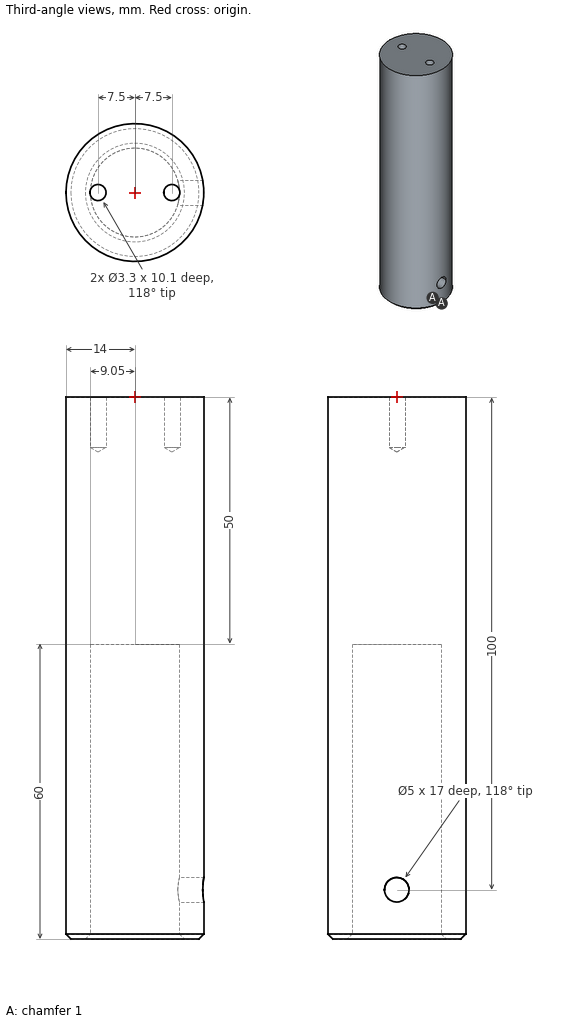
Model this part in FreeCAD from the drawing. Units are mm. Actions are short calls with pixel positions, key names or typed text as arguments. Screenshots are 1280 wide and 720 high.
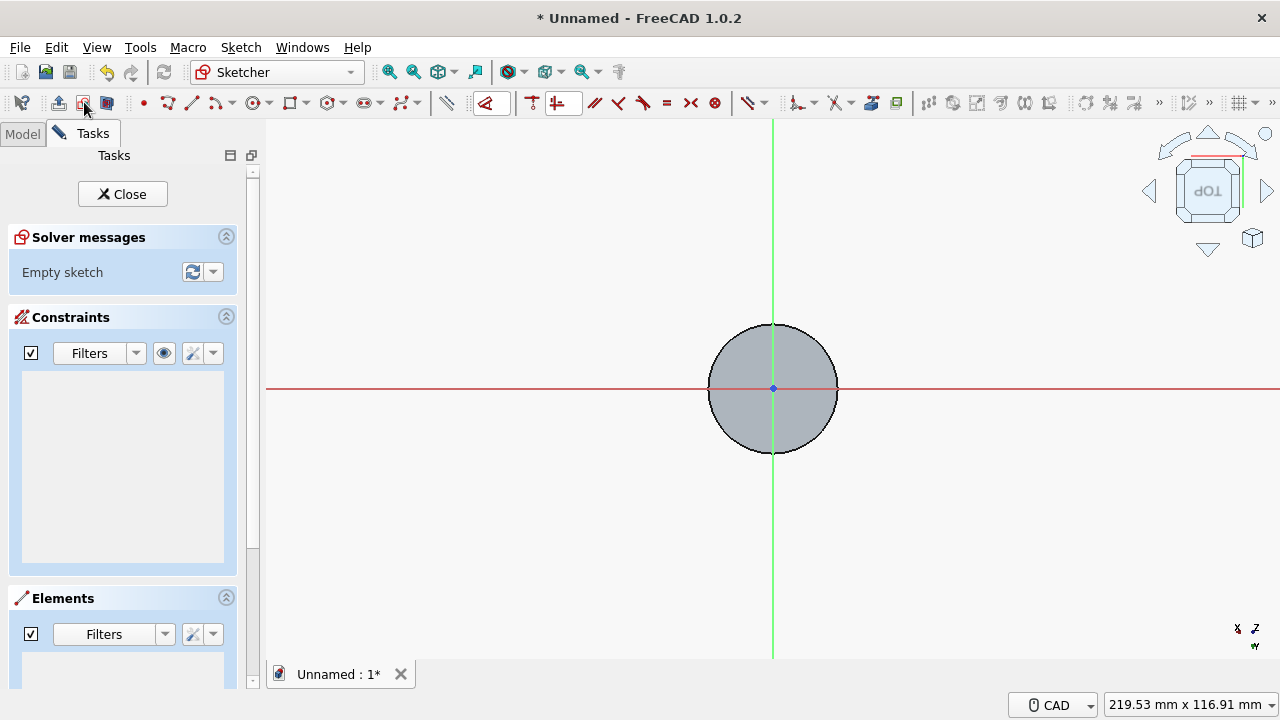
scroll(784, 389, up, 10)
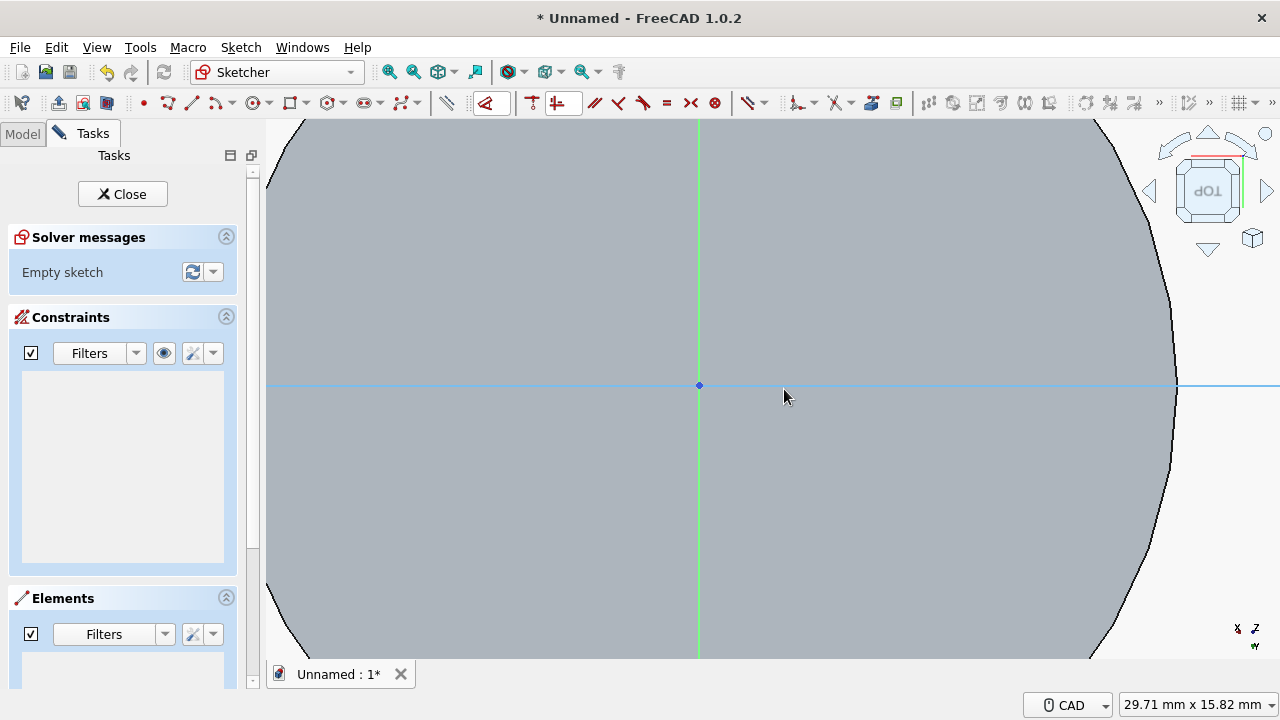
click(254, 104)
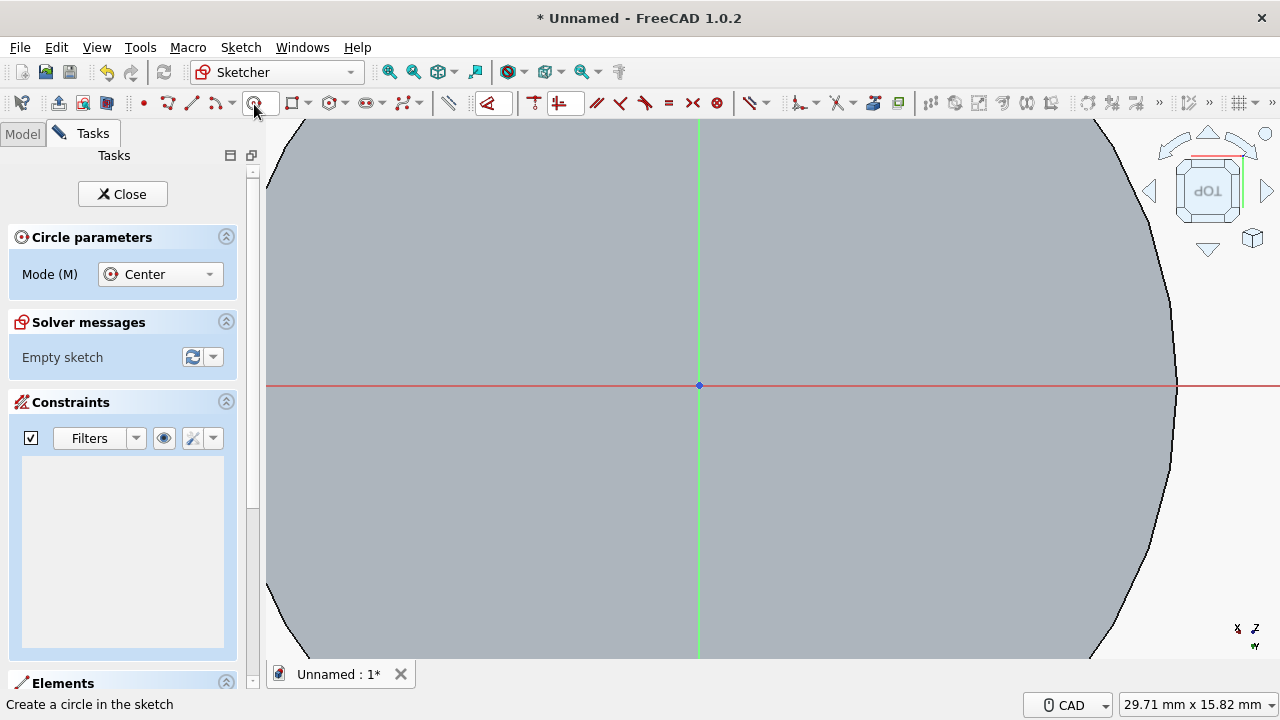
click(955, 386)
click(995, 346)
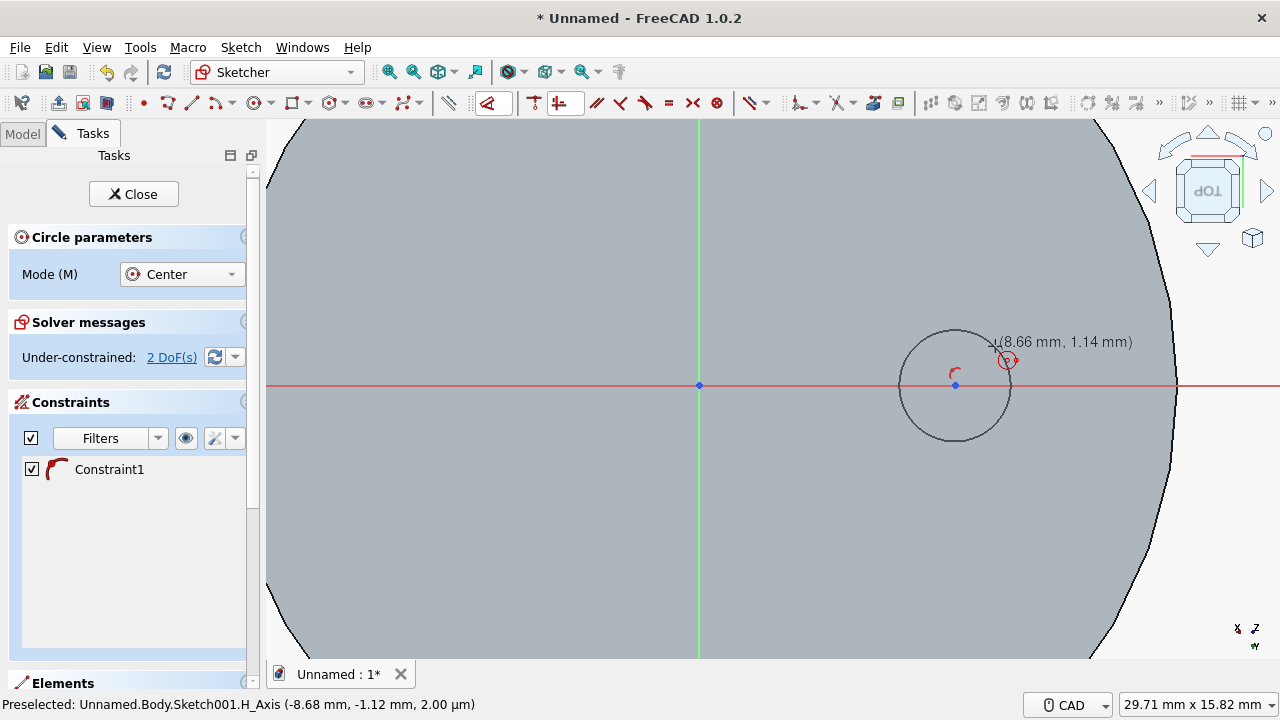
click(443, 386)
click(483, 346)
key(Escape)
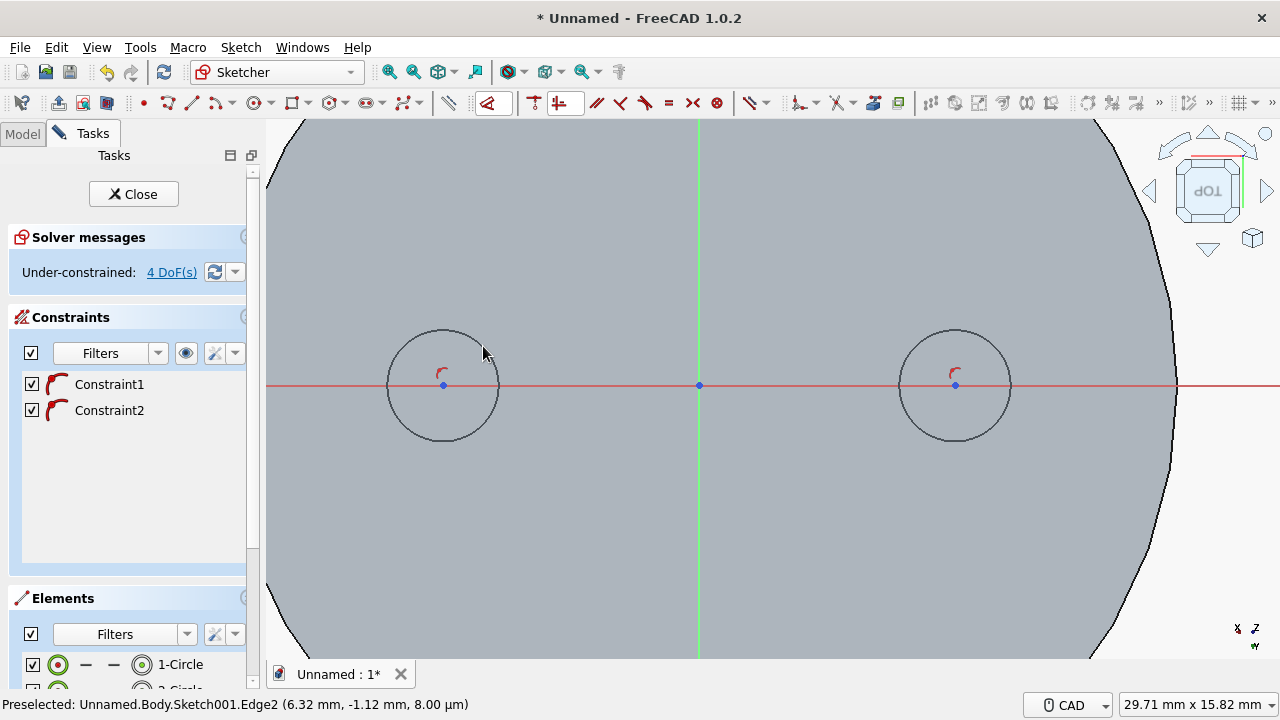
click(994, 346)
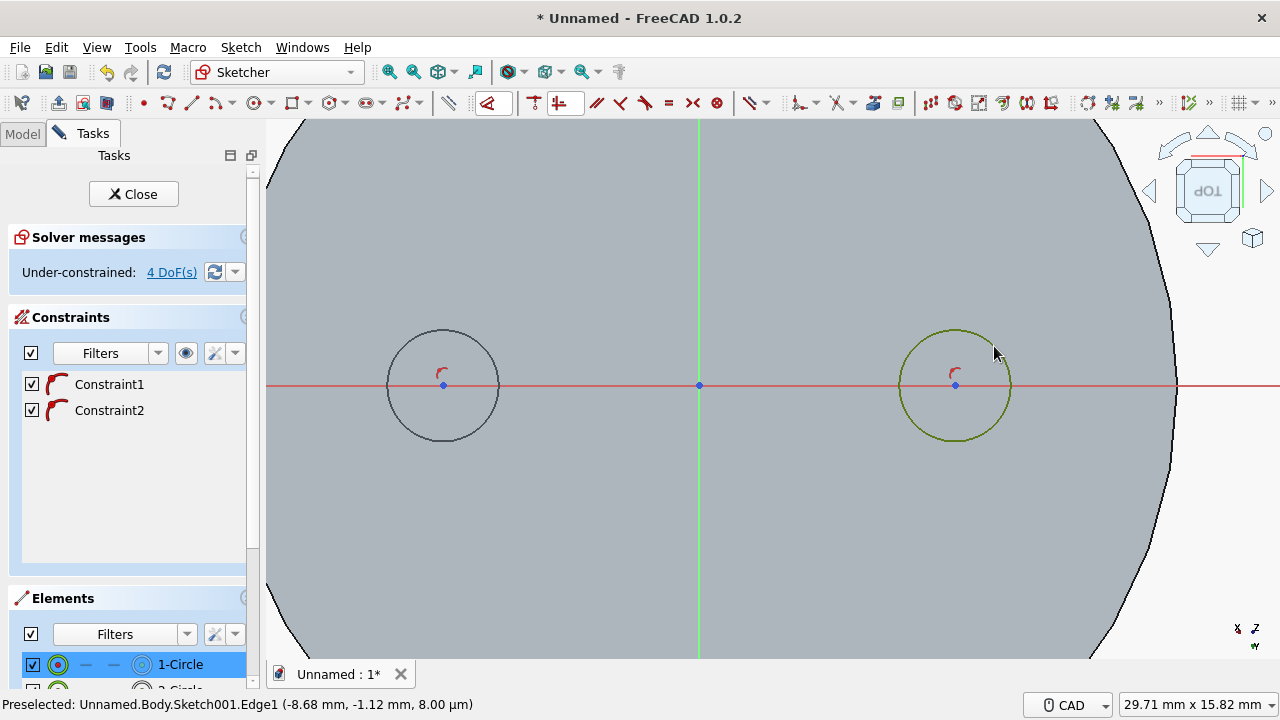
click(482, 346)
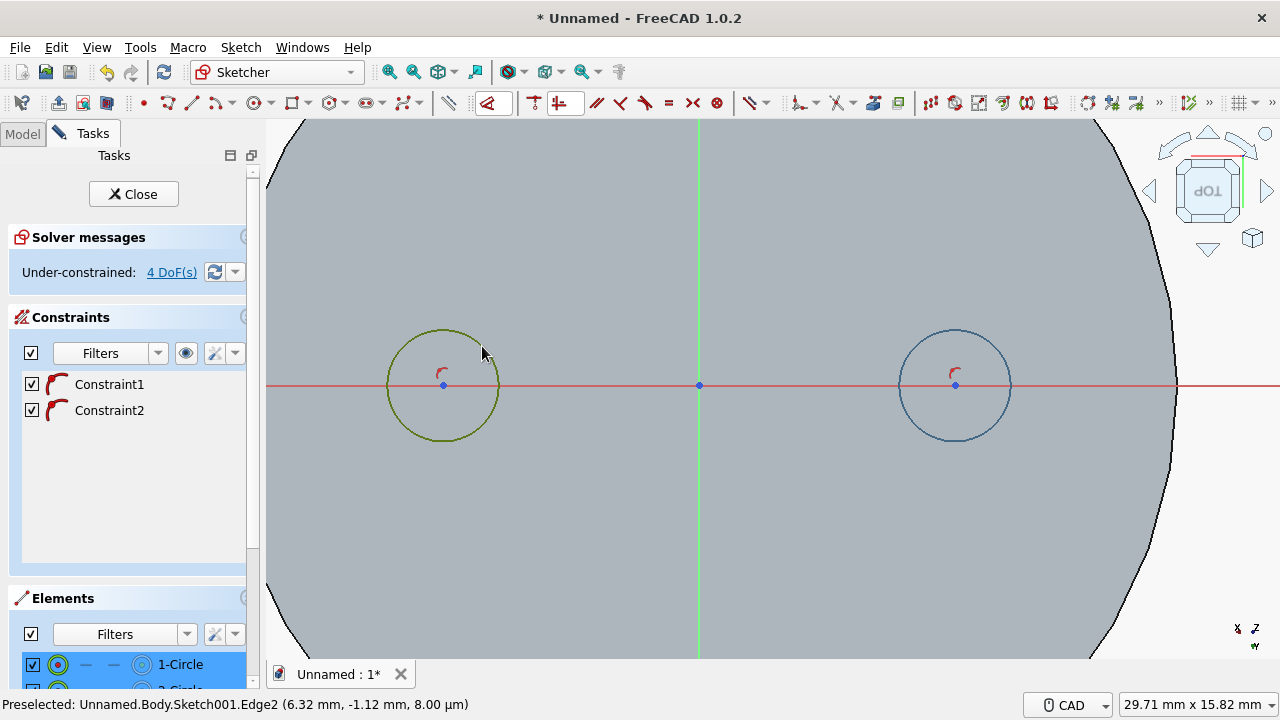
click(670, 104)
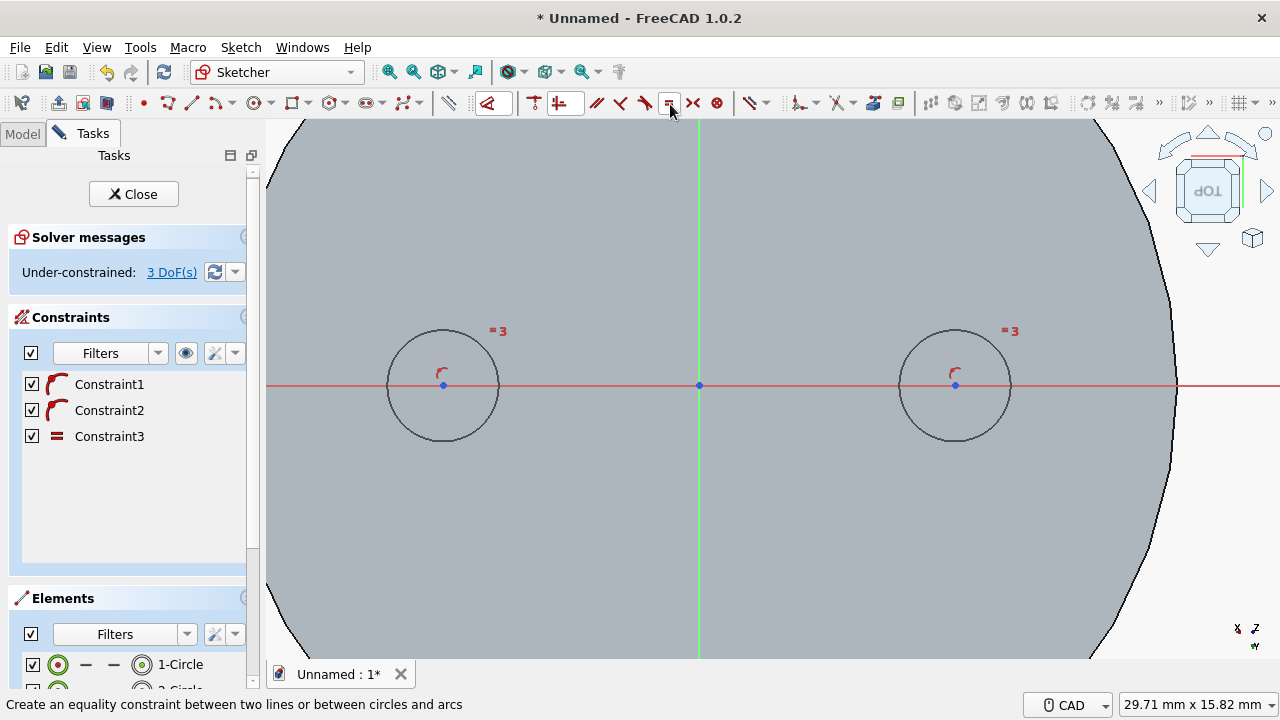
click(994, 346)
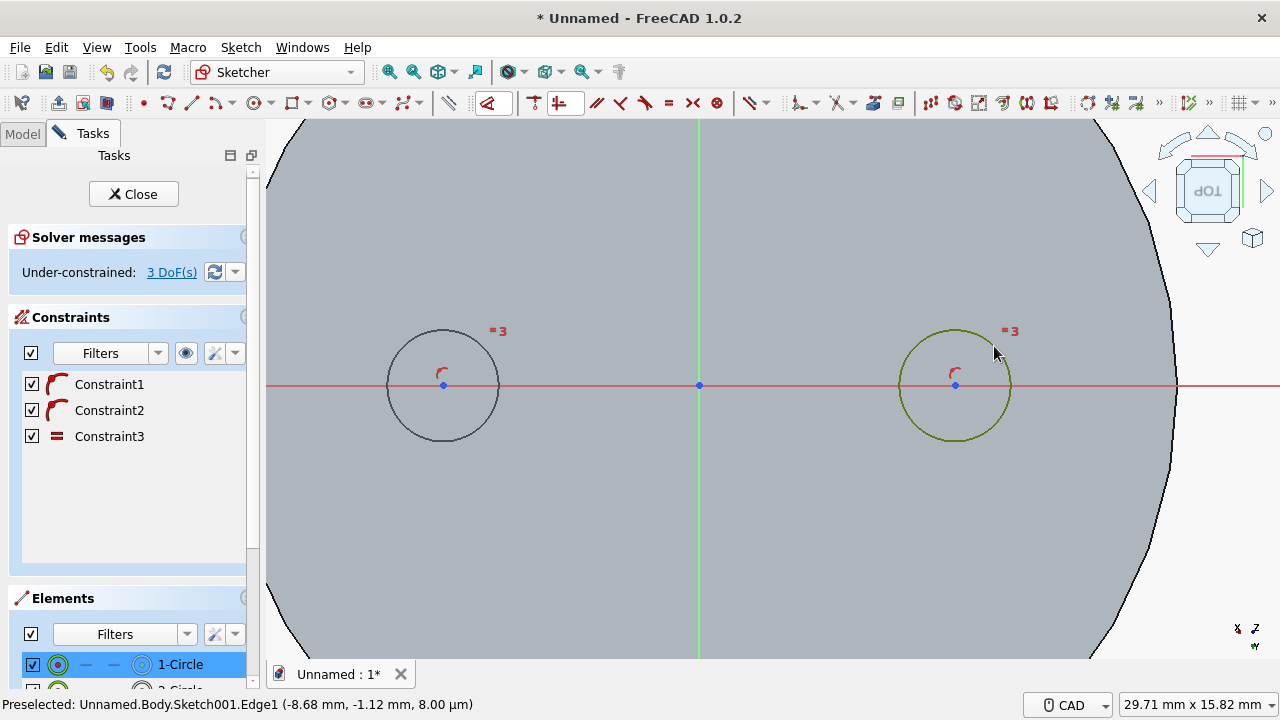
click(506, 104)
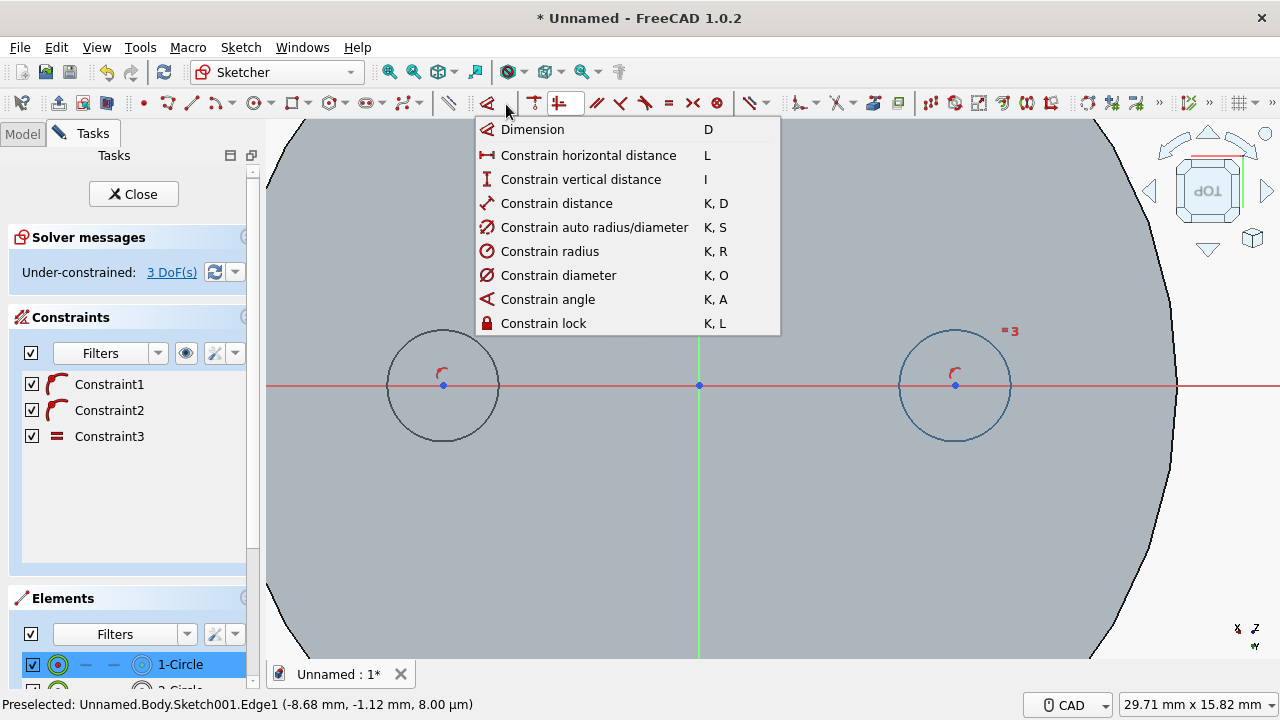
click(628, 275)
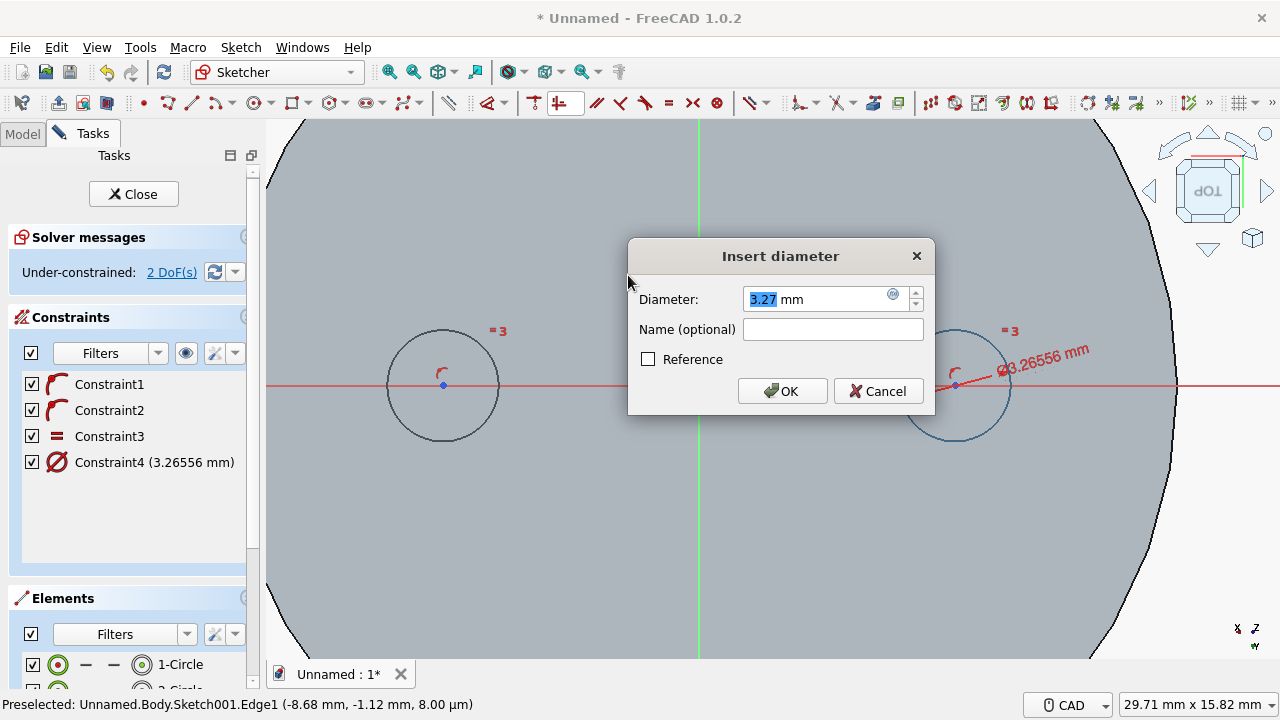
text(3.3)
key(Return)